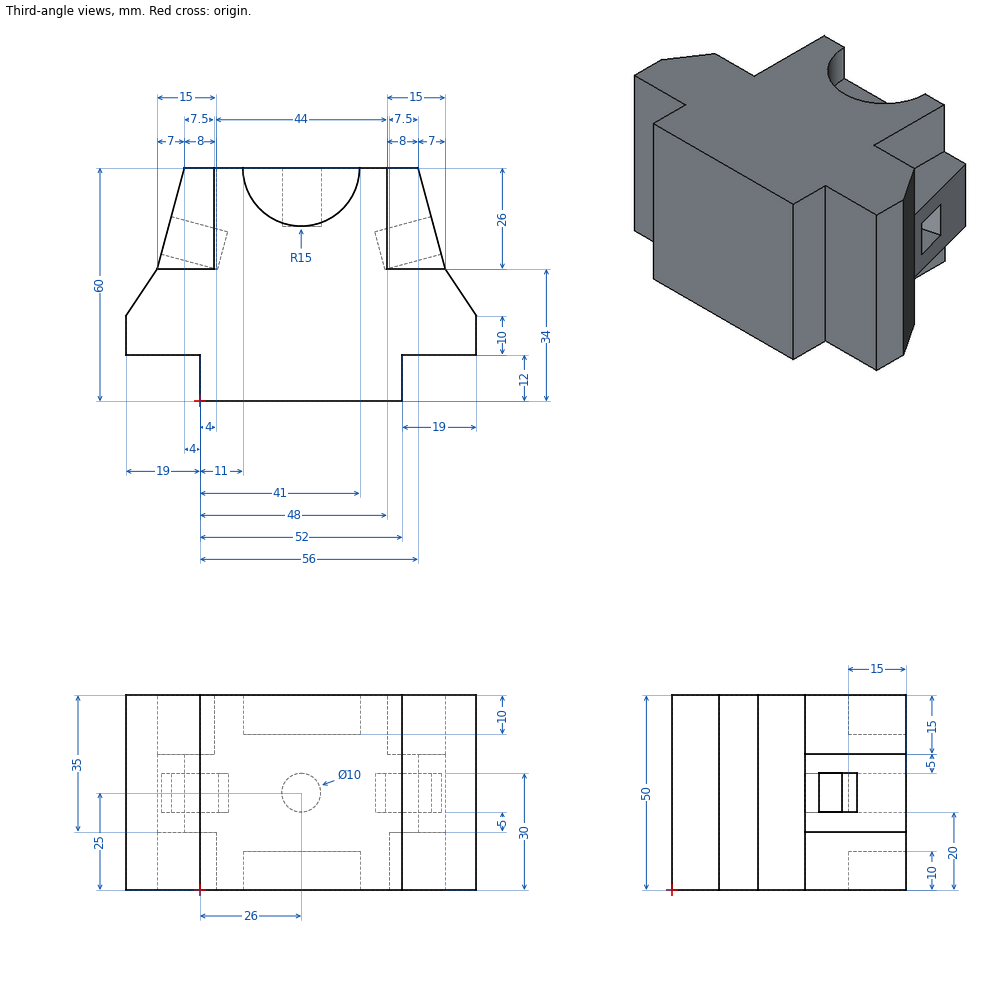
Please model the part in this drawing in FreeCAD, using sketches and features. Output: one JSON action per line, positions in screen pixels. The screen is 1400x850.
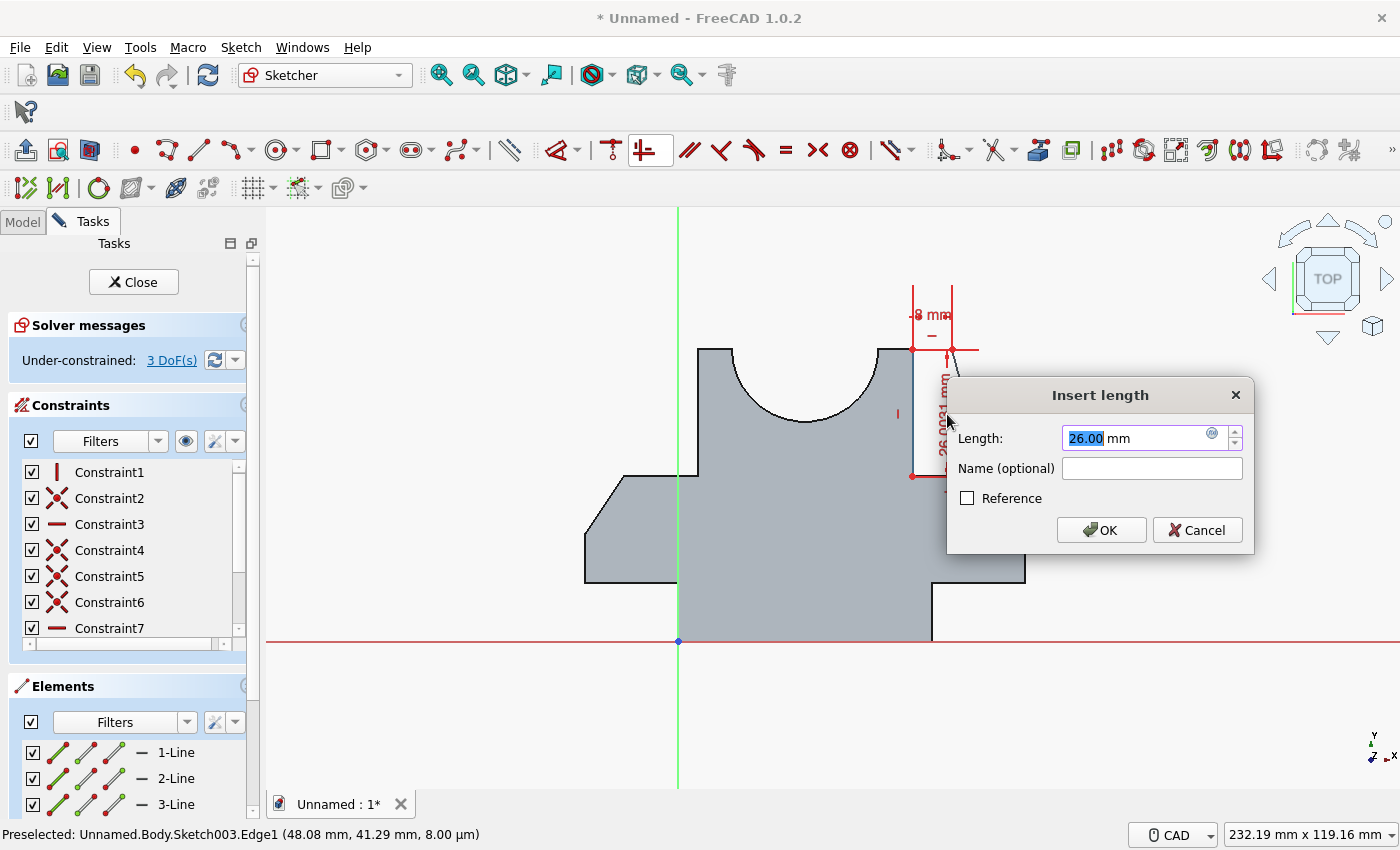
{"action": "type", "text": "26"}
{"action": "key", "text": "Return"}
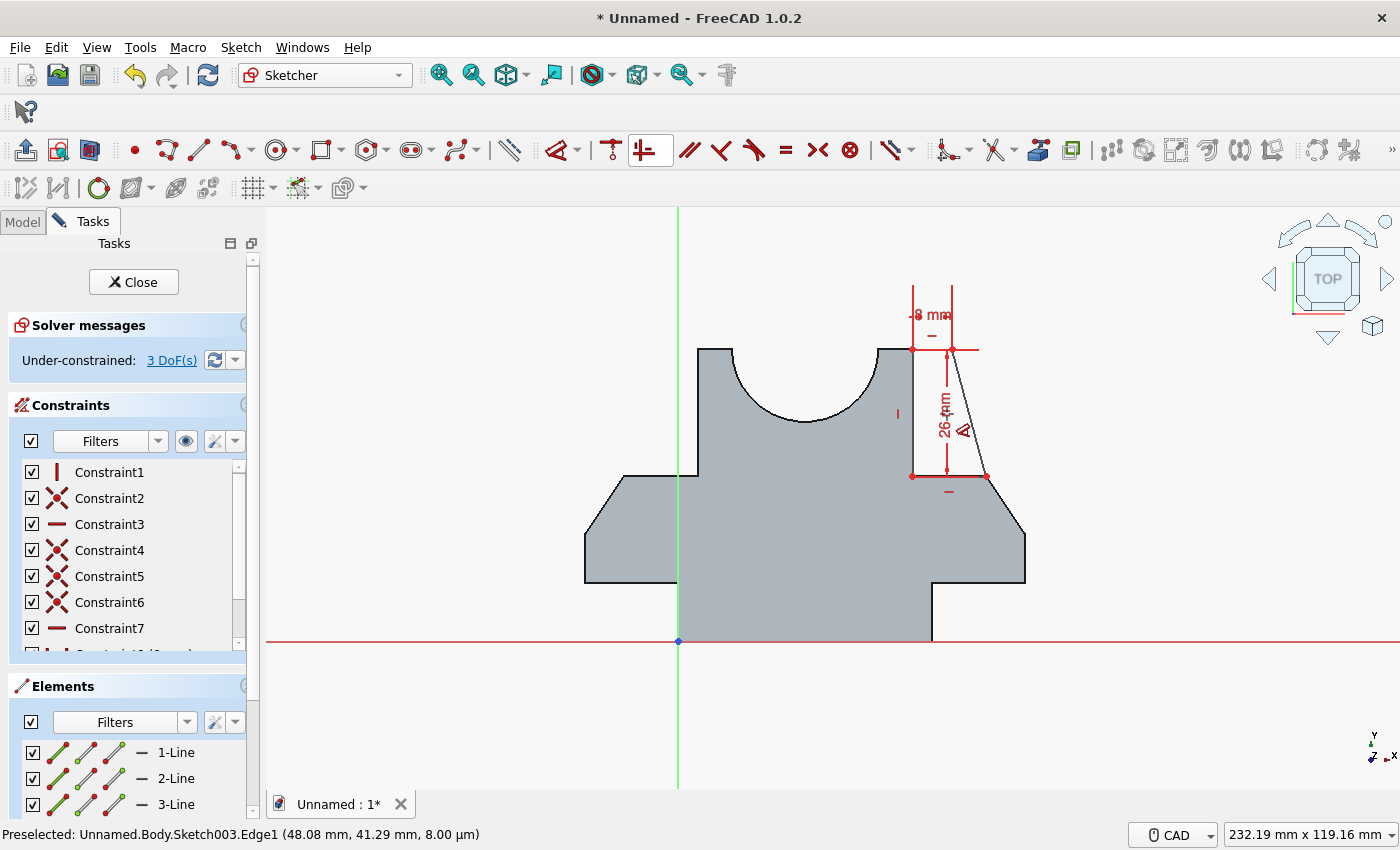
{"action": "left_click", "coordinate": [964, 477]}
{"action": "left_click", "coordinate": [949, 443]}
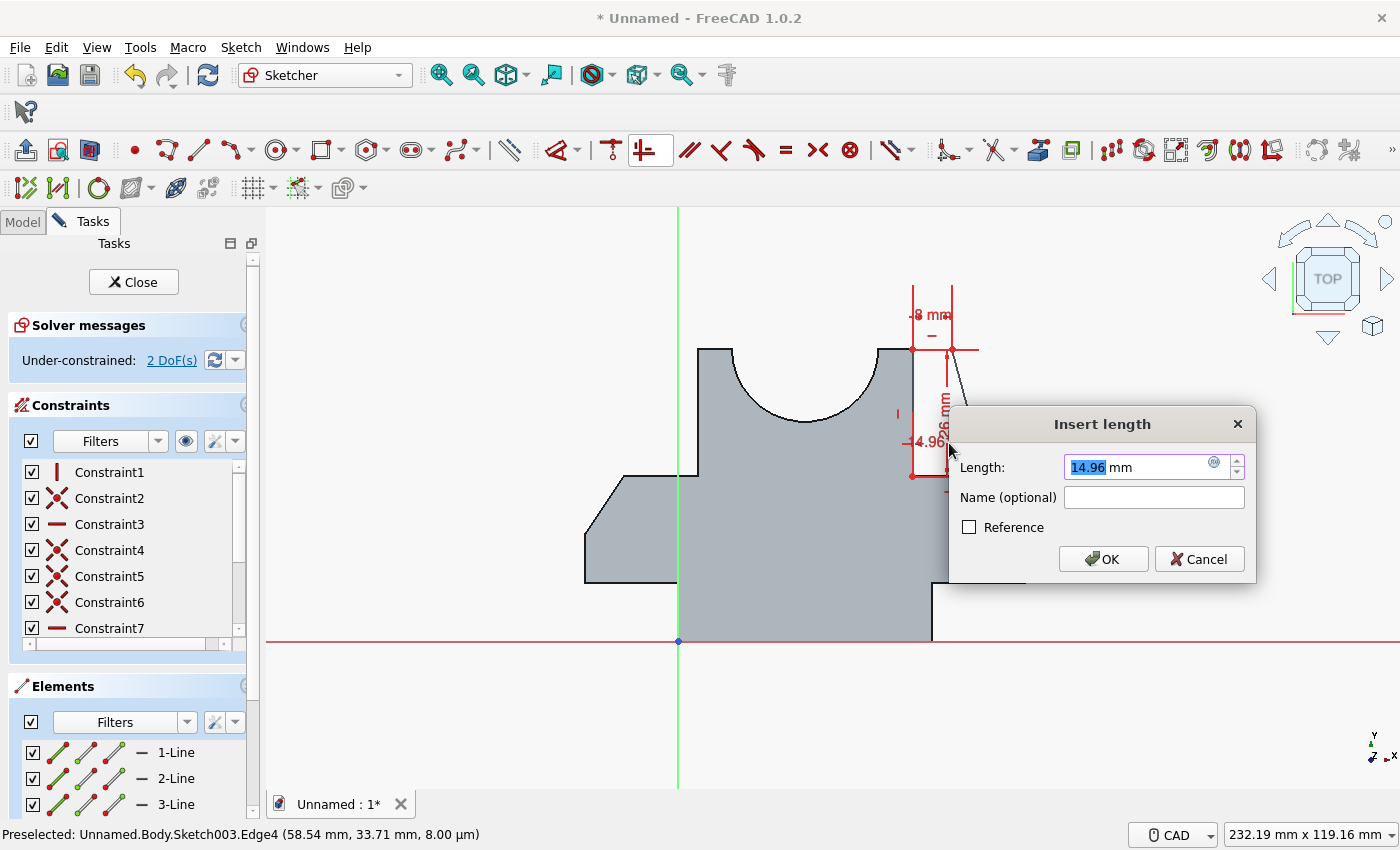
{"action": "type", "text": "15"}
{"action": "key", "text": "Return"}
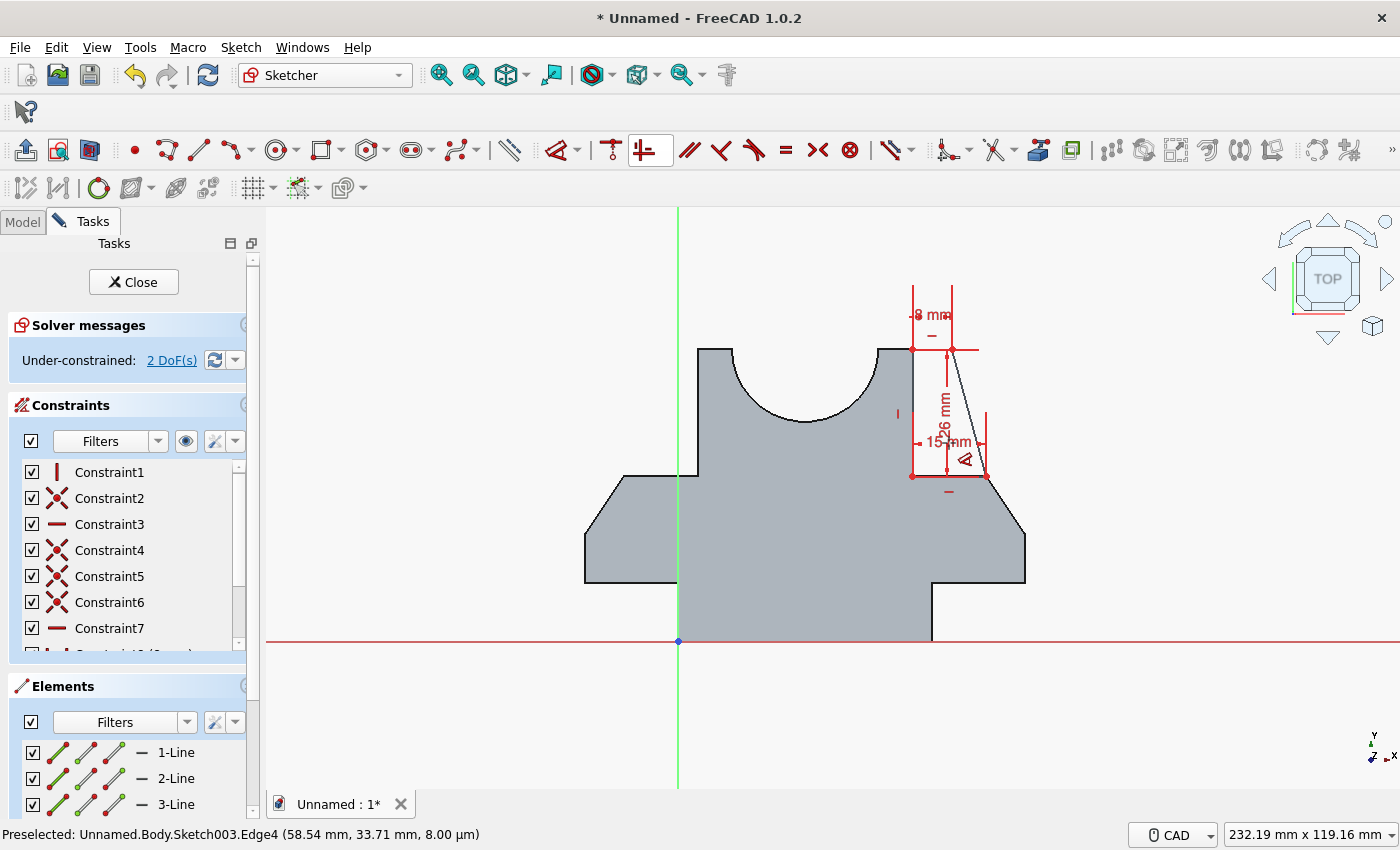
{"action": "left_click", "coordinate": [913, 477]}
{"action": "left_click", "coordinate": [796, 676]}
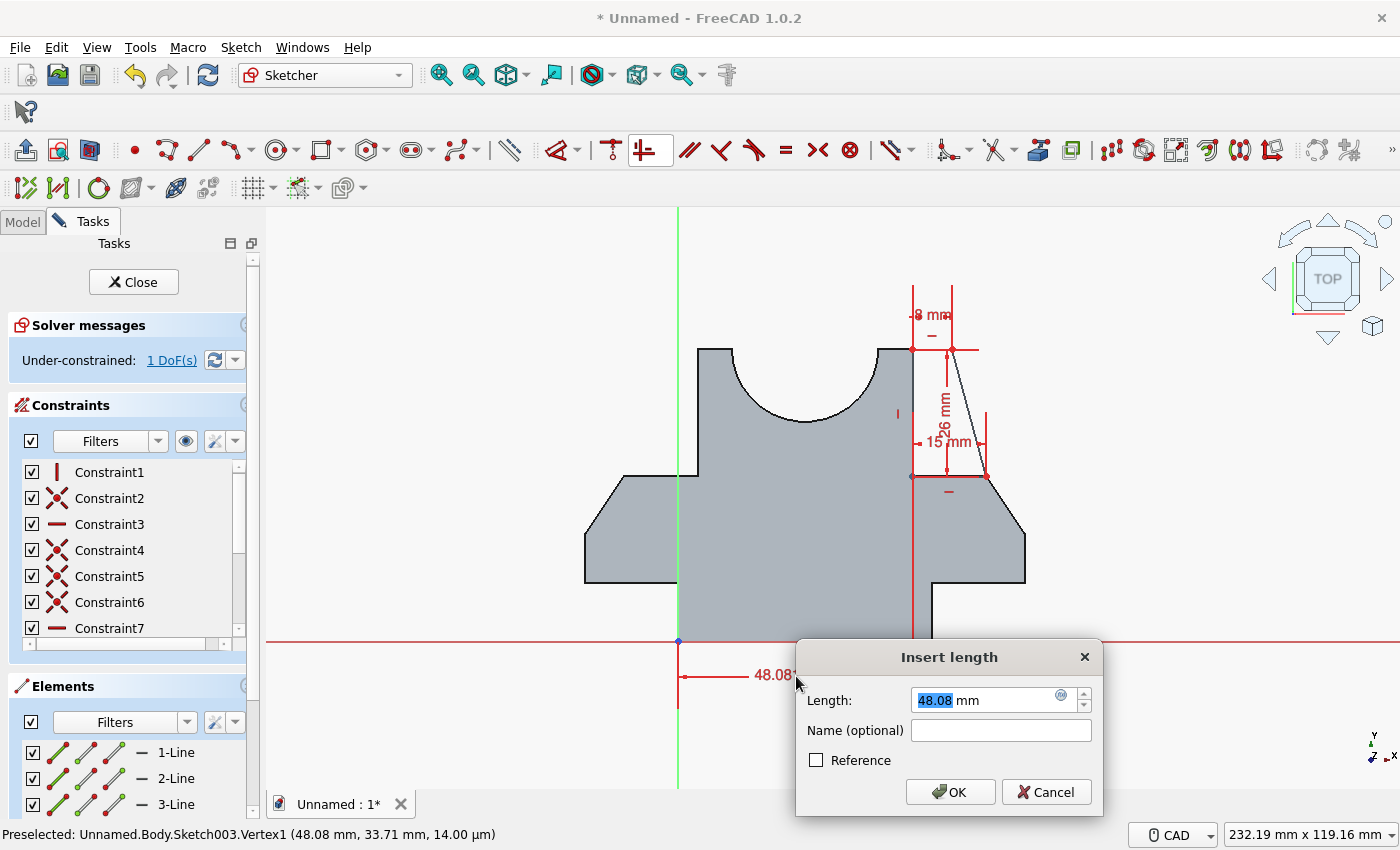
{"action": "type", "text": "48"}
{"action": "key", "text": "Return"}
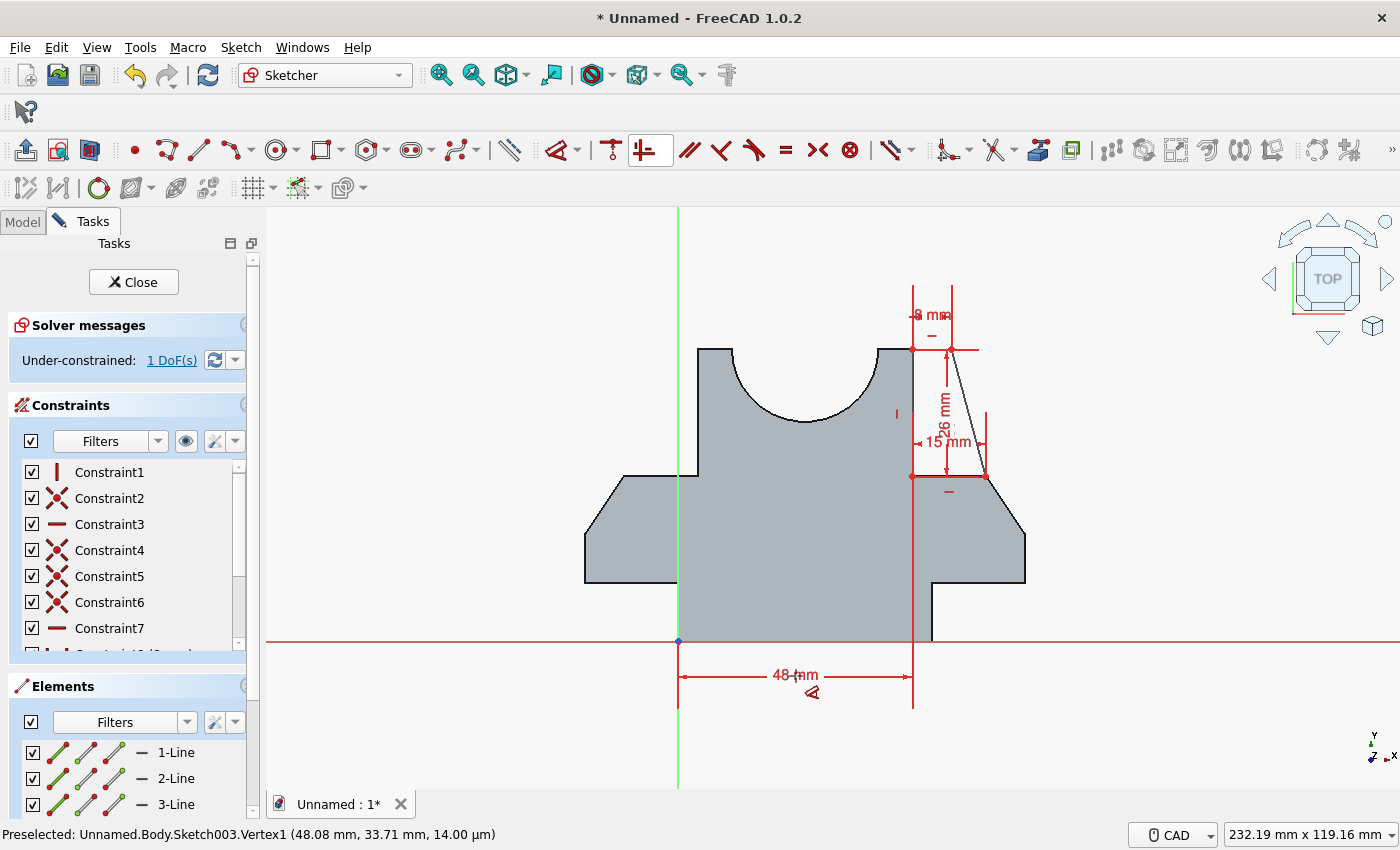
{"action": "left_click", "coordinate": [913, 477]}
{"action": "left_click", "coordinate": [644, 559]}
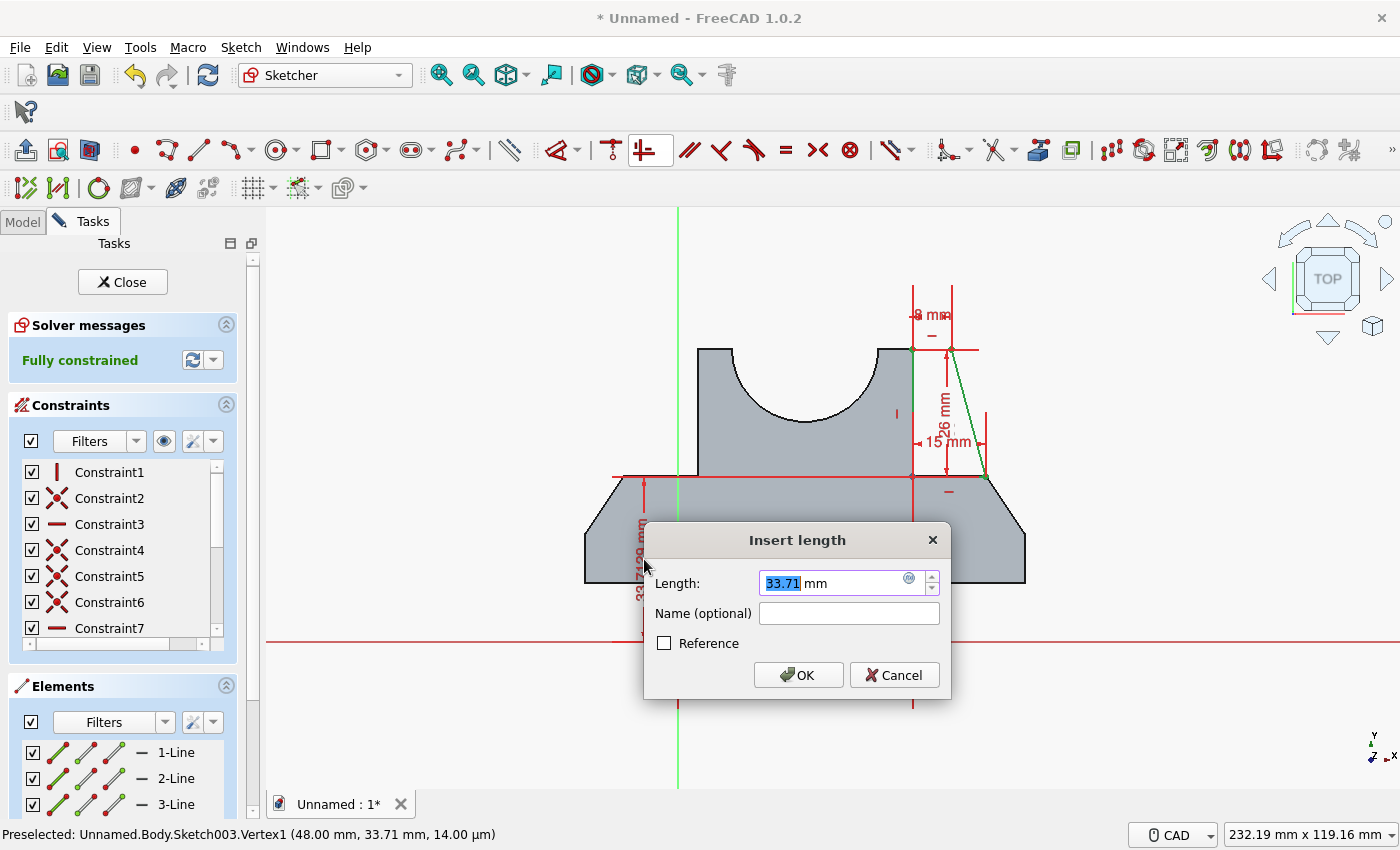
{"action": "type", "text": "34"}
{"action": "key", "text": "Return"}
{"action": "key", "text": "Escape"}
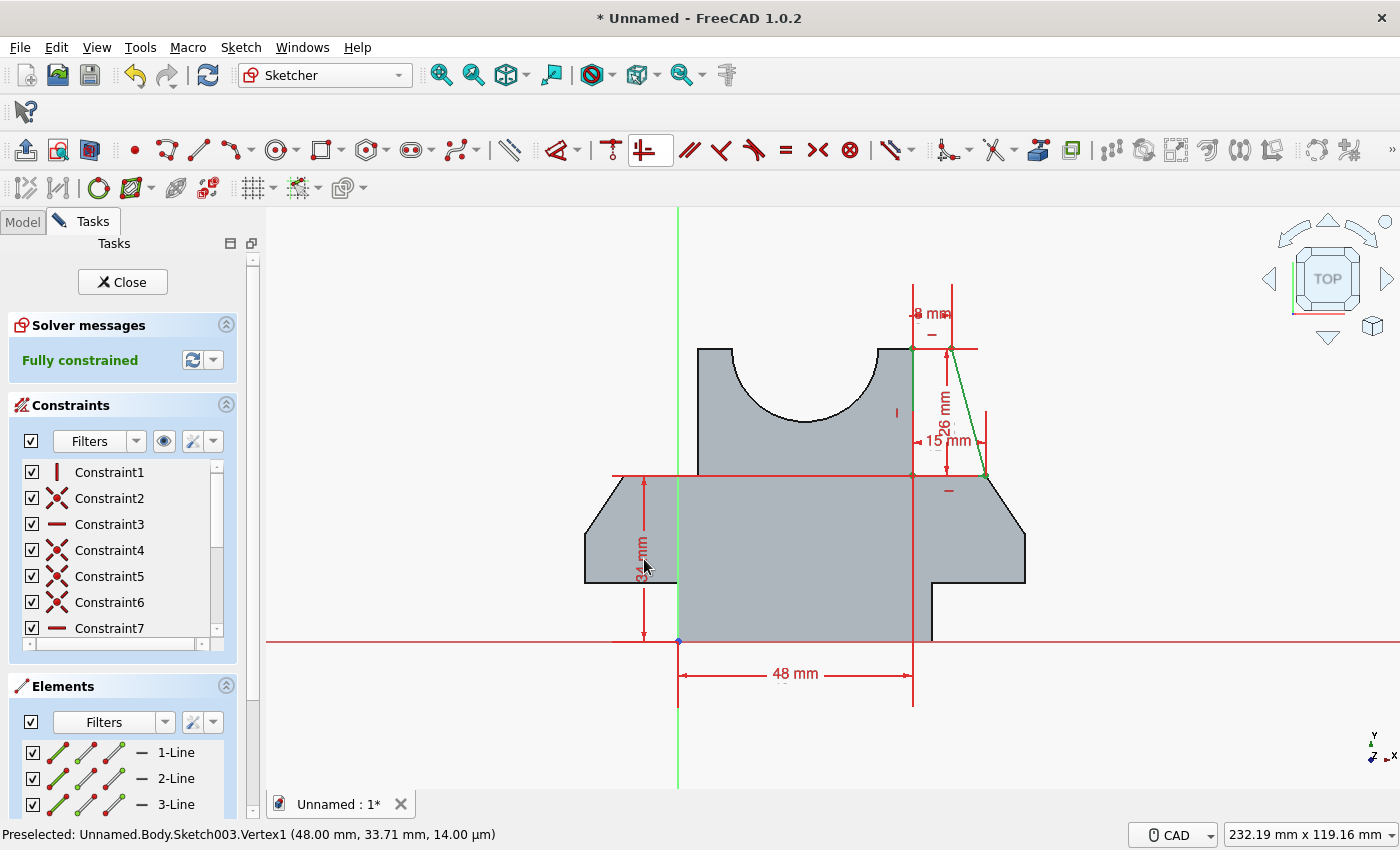
{"action": "left_click", "coordinate": [123, 282]}